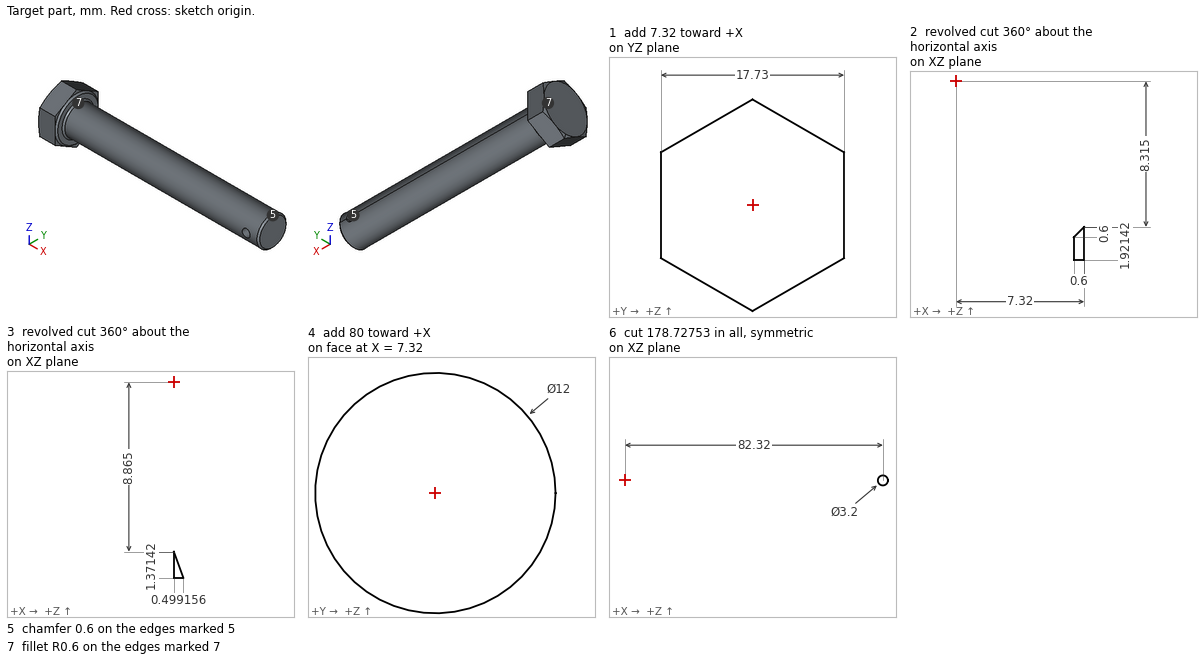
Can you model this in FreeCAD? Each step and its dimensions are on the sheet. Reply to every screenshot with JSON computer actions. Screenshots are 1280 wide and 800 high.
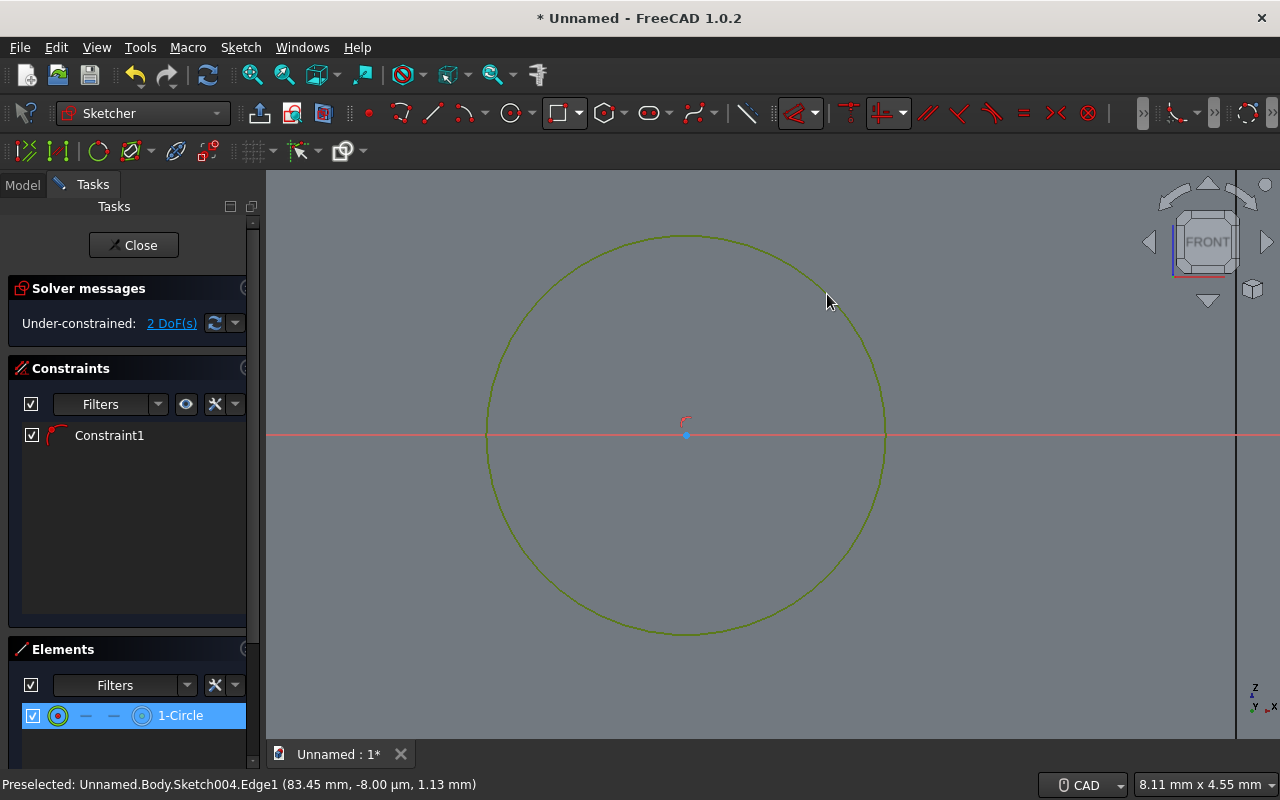
{"action": "key", "text": "k o"}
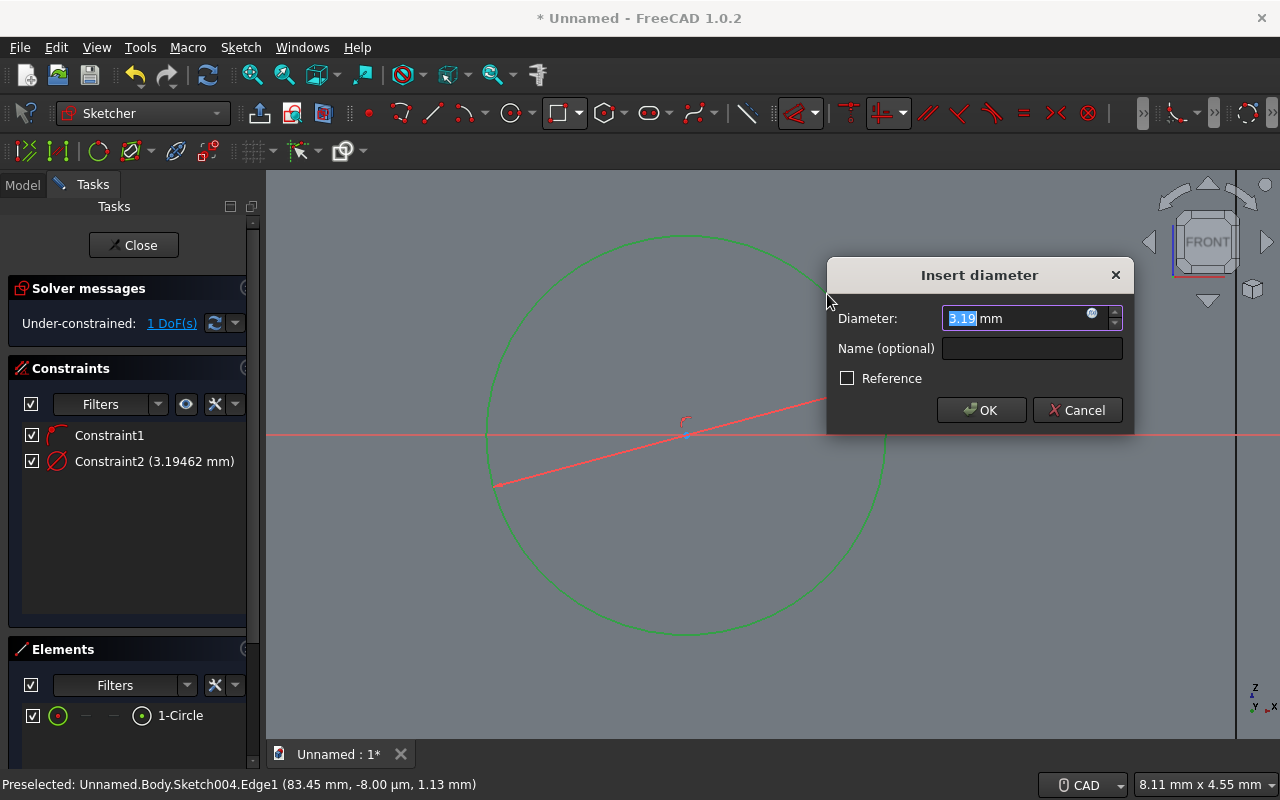
{"action": "type", "text": "3.2"}
{"action": "key", "text": "Return"}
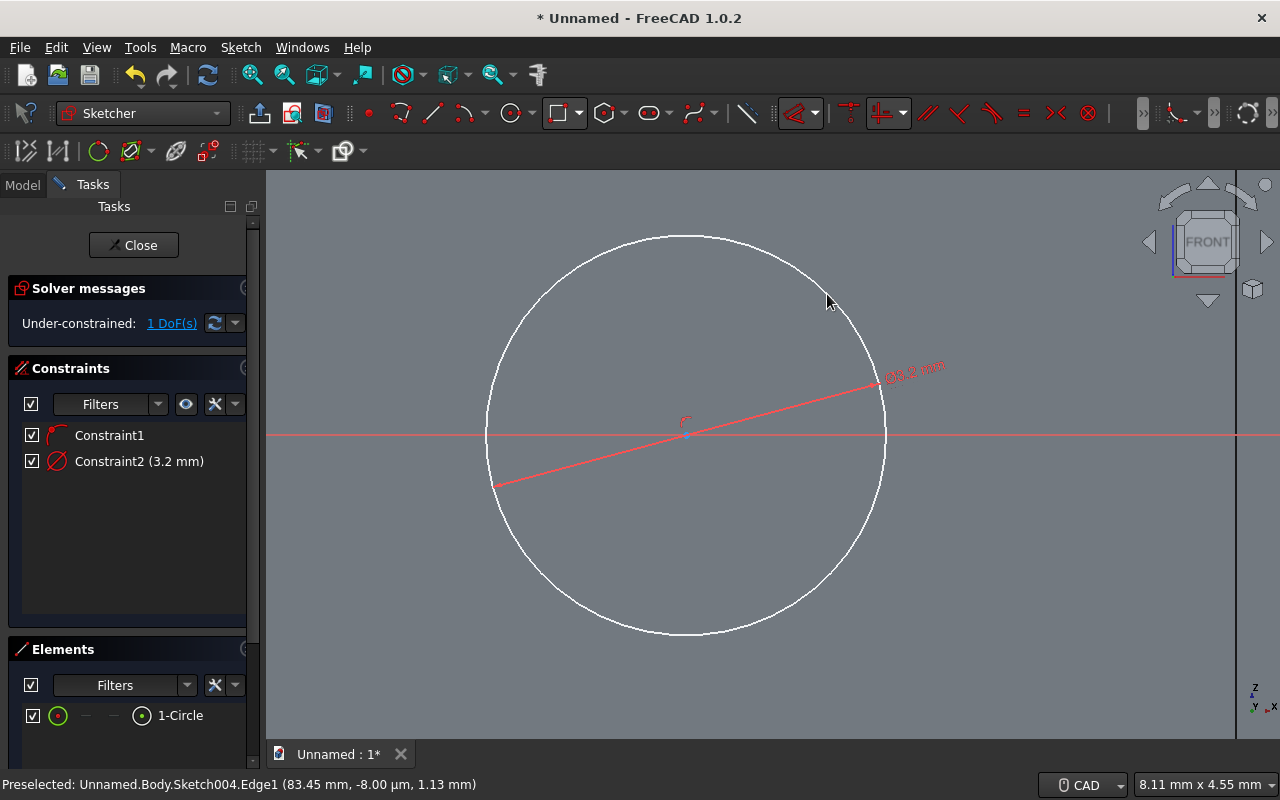
{"action": "left_click", "coordinate": [686, 435]}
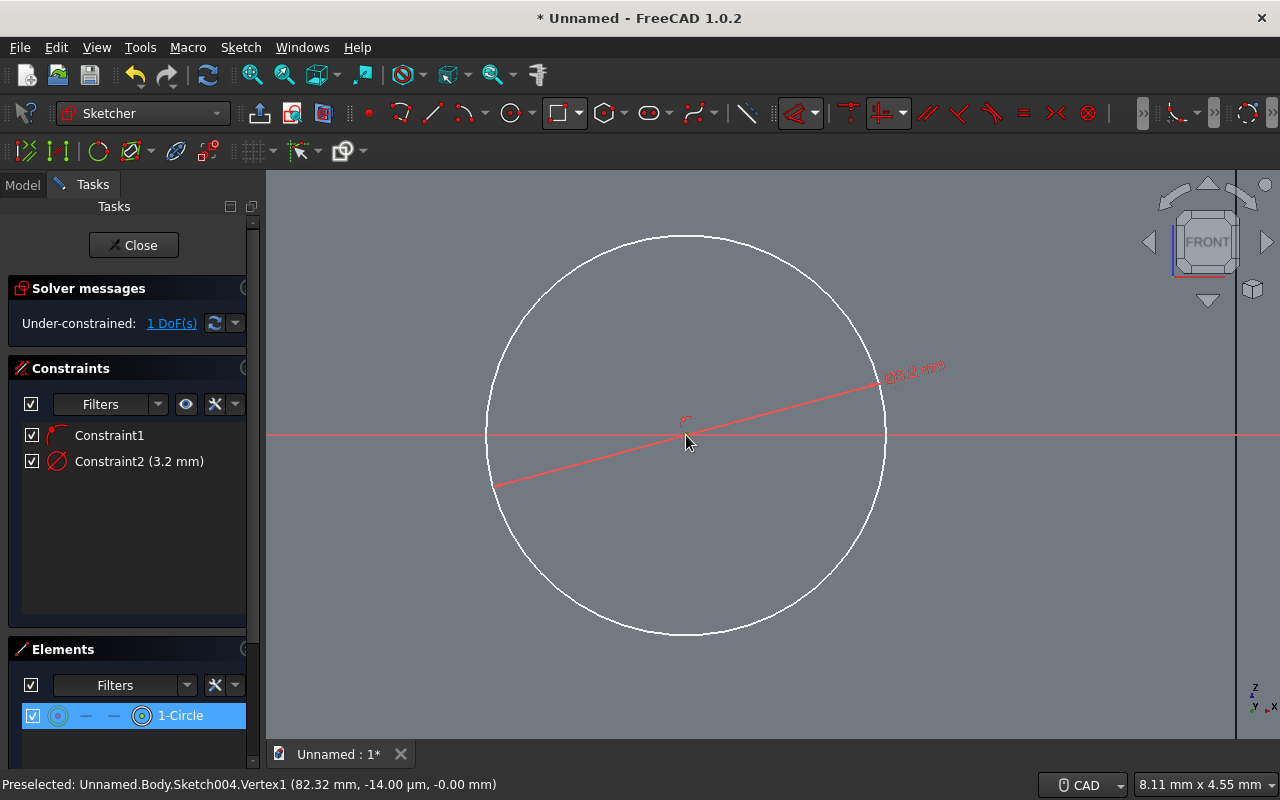
{"action": "key", "text": "l"}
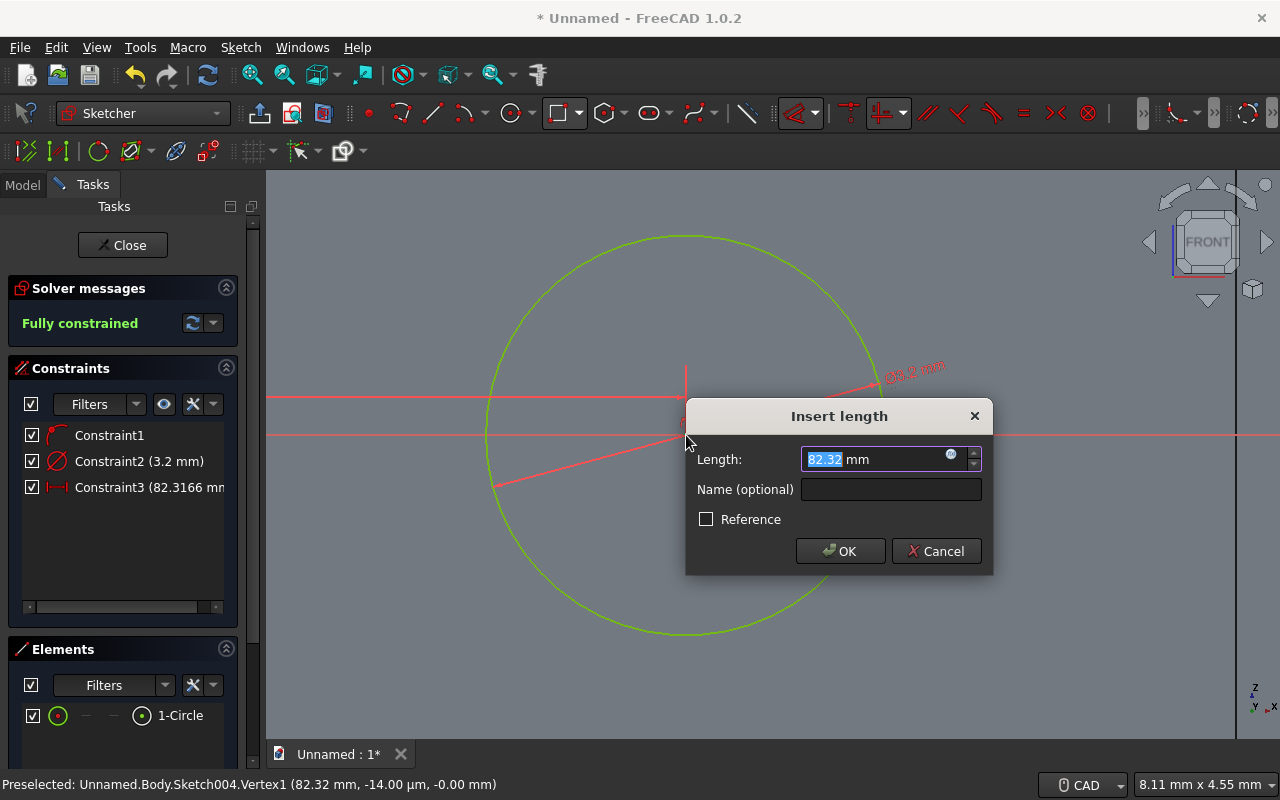
{"action": "type", "text": "82.32"}
{"action": "key", "text": "Return"}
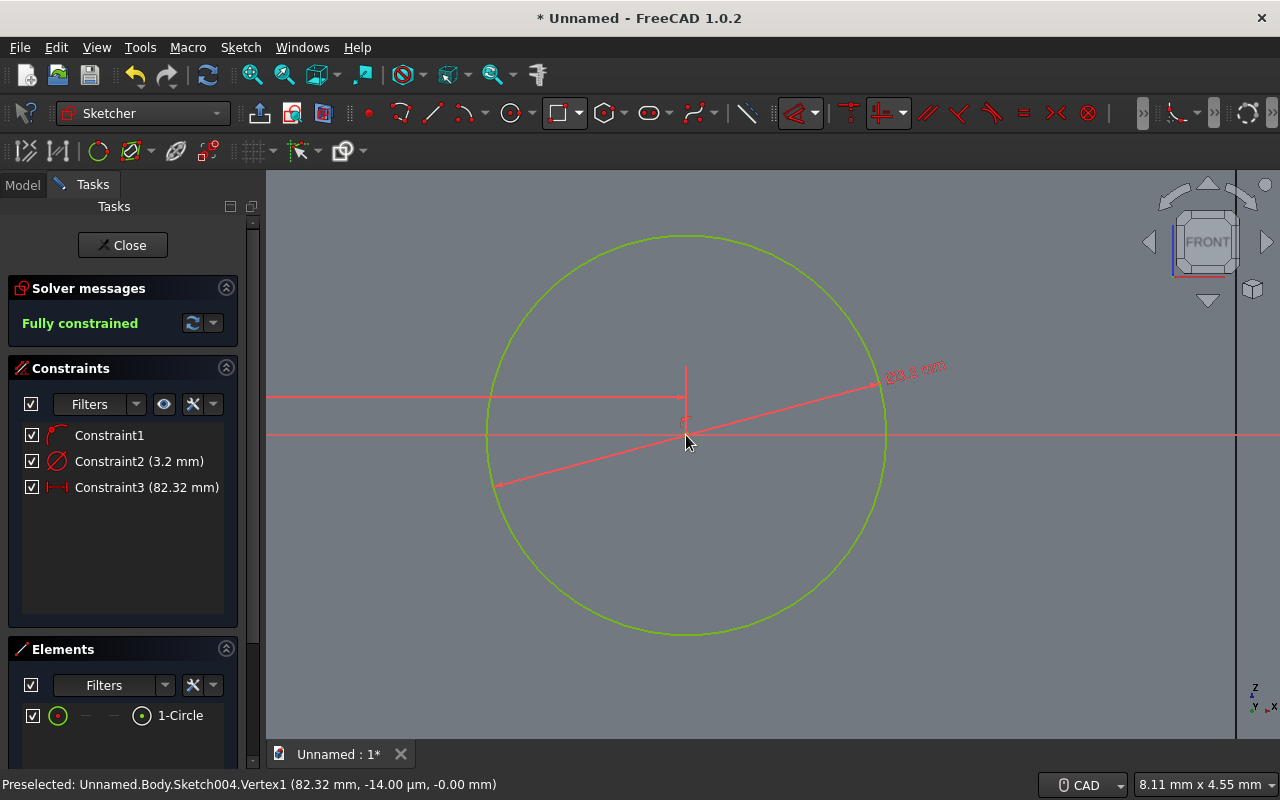
{"action": "left_click", "coordinate": [123, 245]}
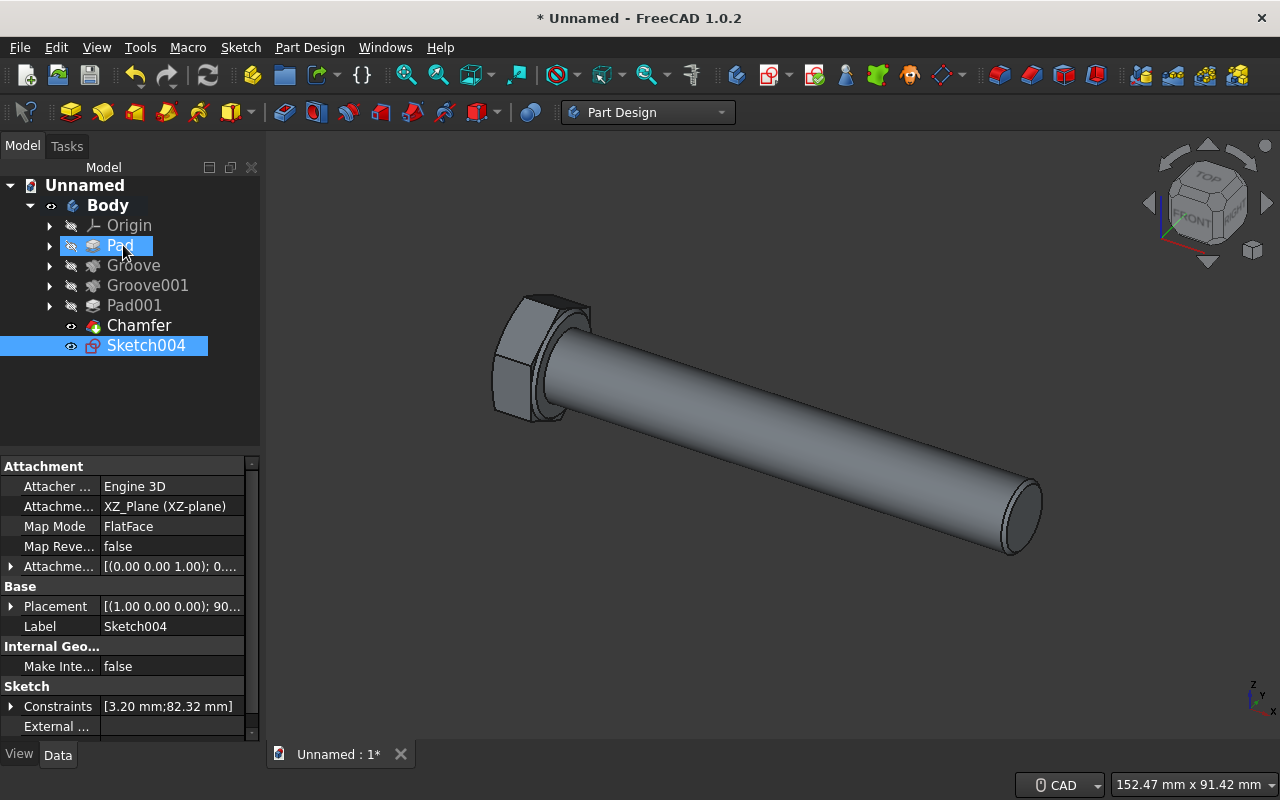
{"action": "left_click", "coordinate": [286, 112]}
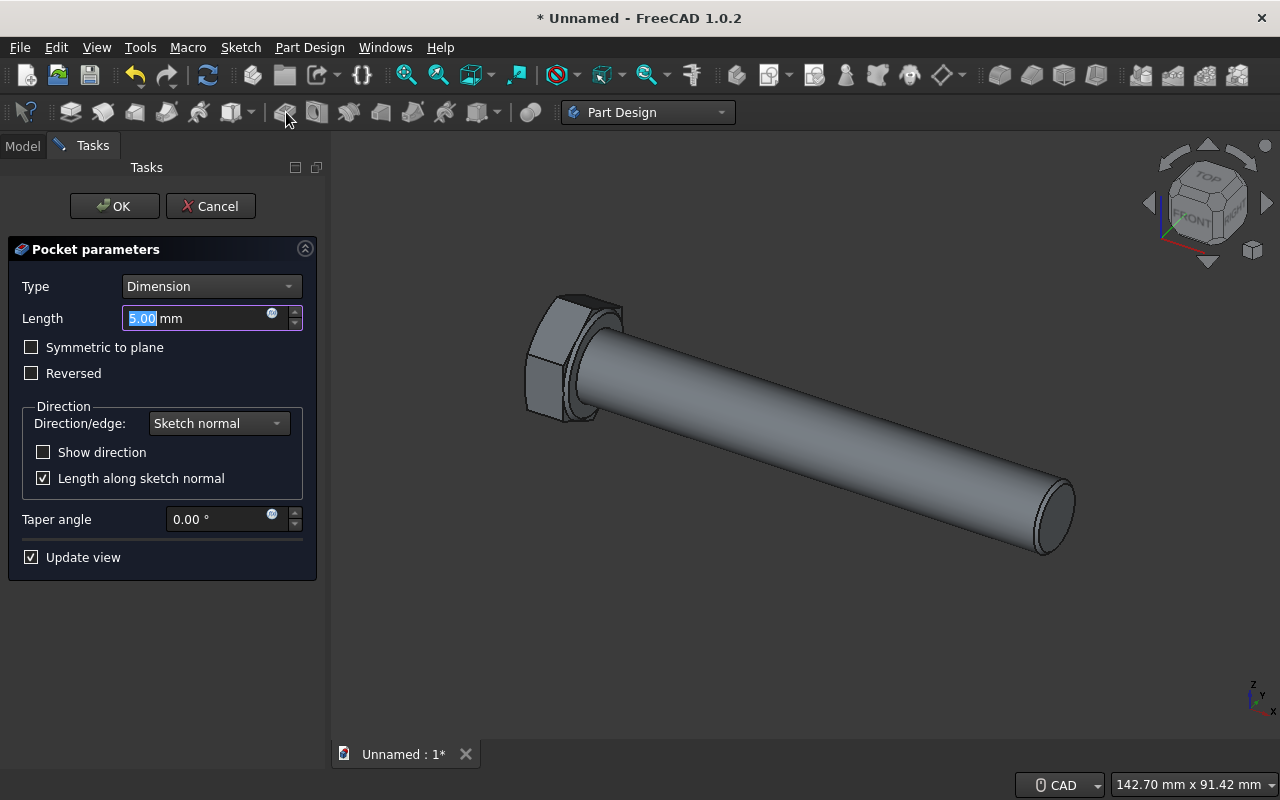
{"action": "type", "text": "178.72753"}
{"action": "key", "text": "Tab"}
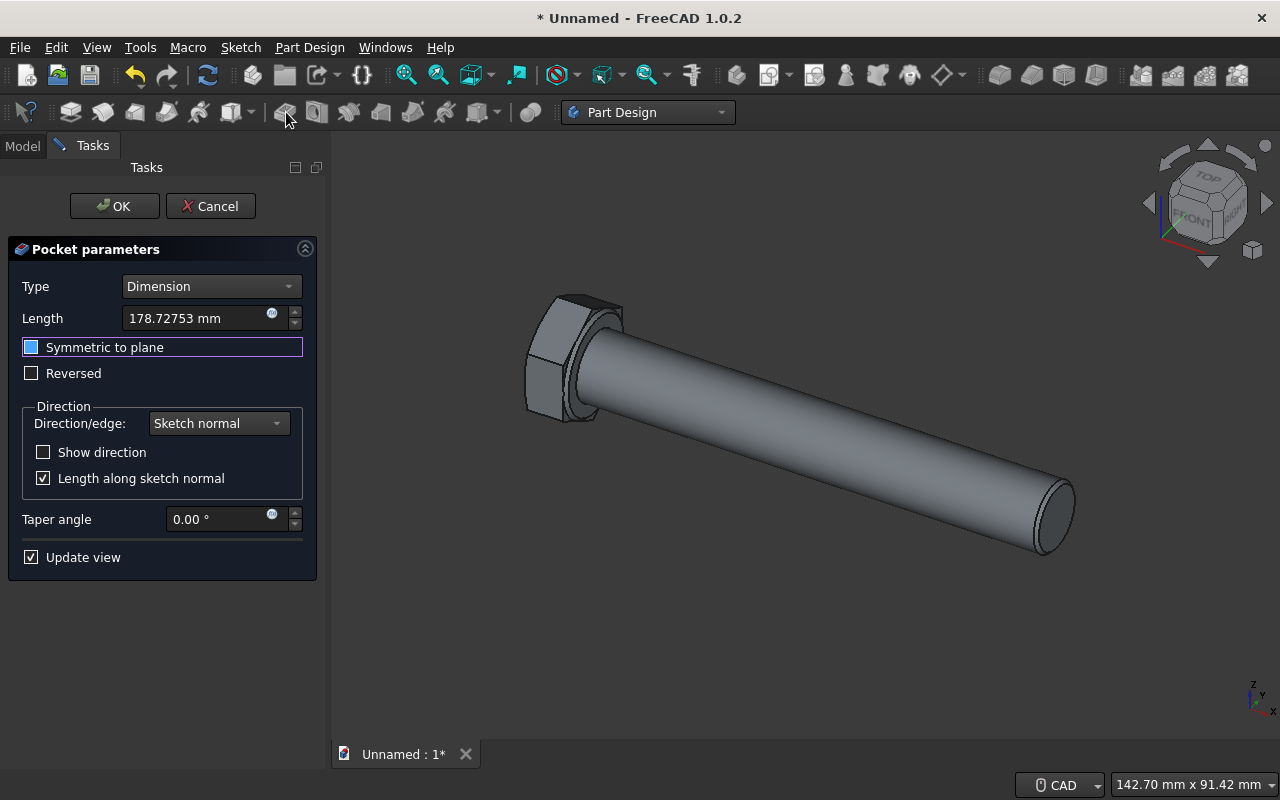
{"action": "left_click", "coordinate": [30, 347]}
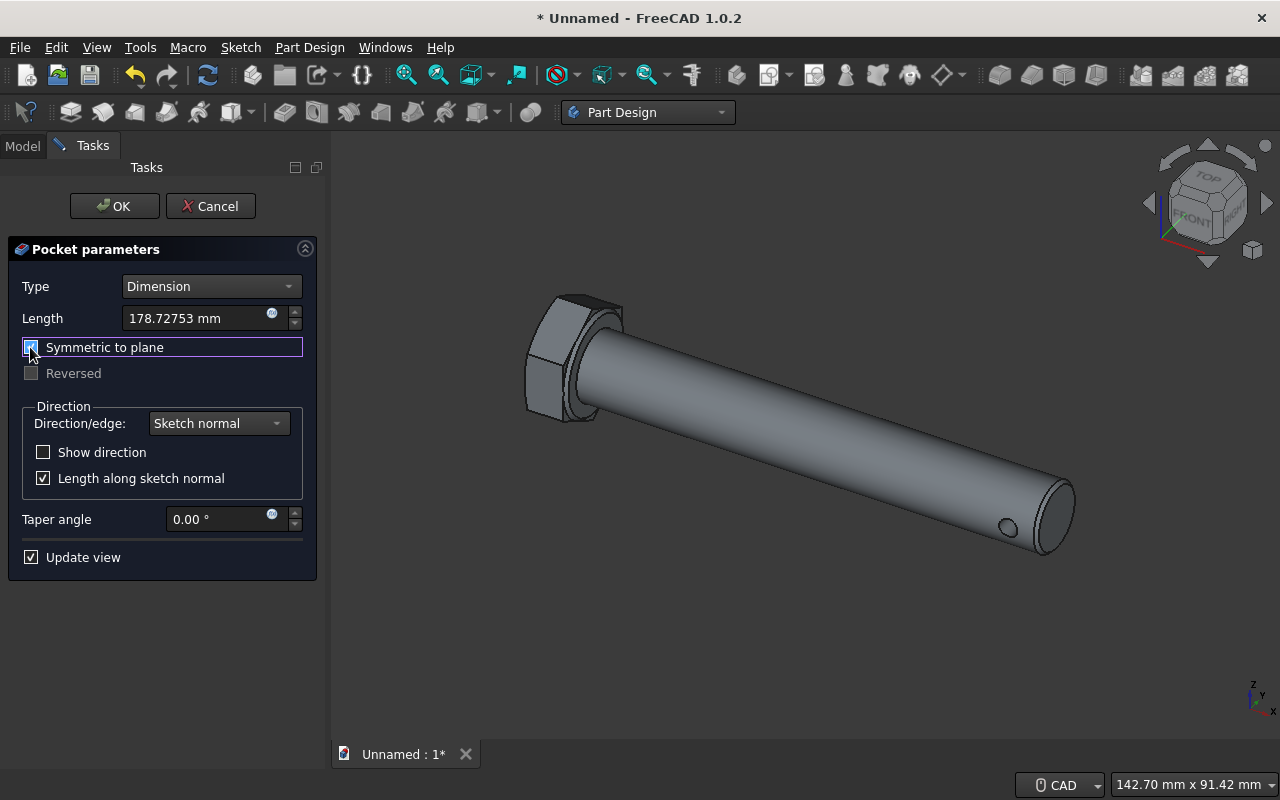
{"action": "left_click", "coordinate": [115, 206]}